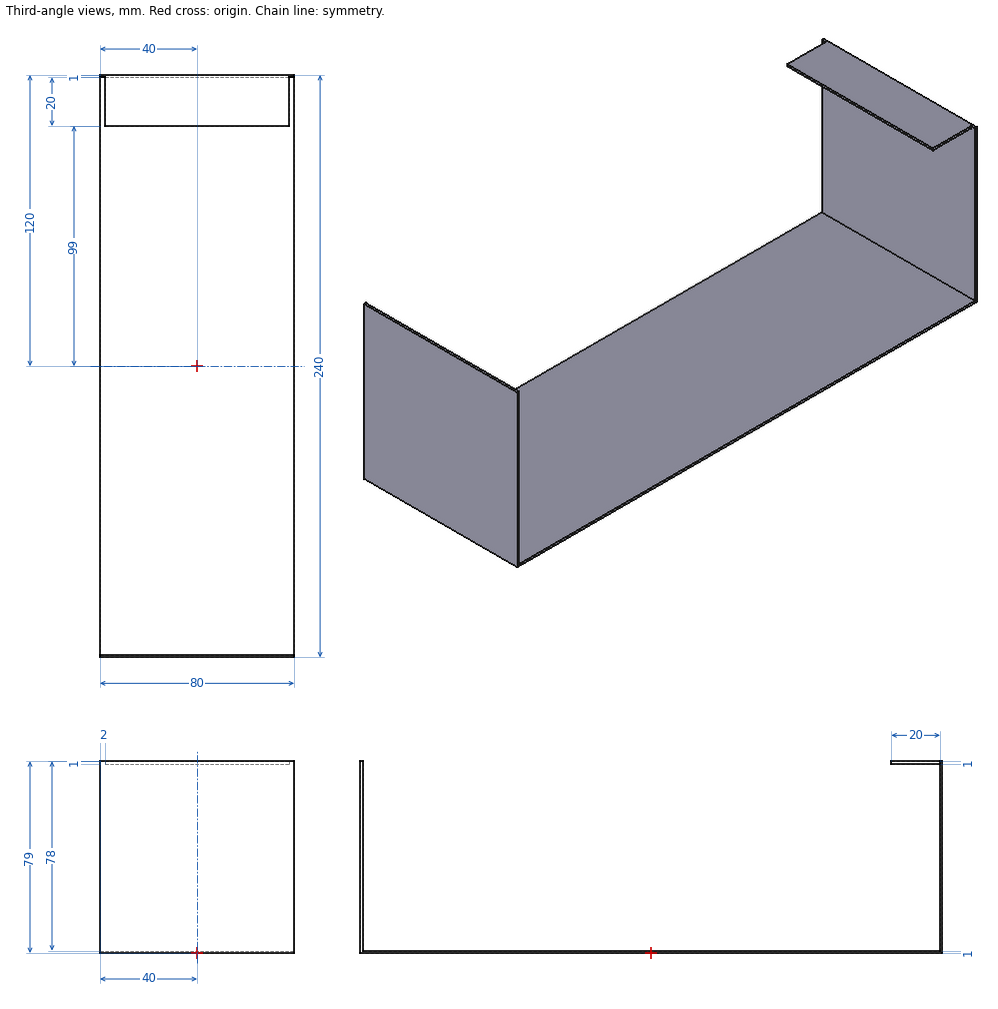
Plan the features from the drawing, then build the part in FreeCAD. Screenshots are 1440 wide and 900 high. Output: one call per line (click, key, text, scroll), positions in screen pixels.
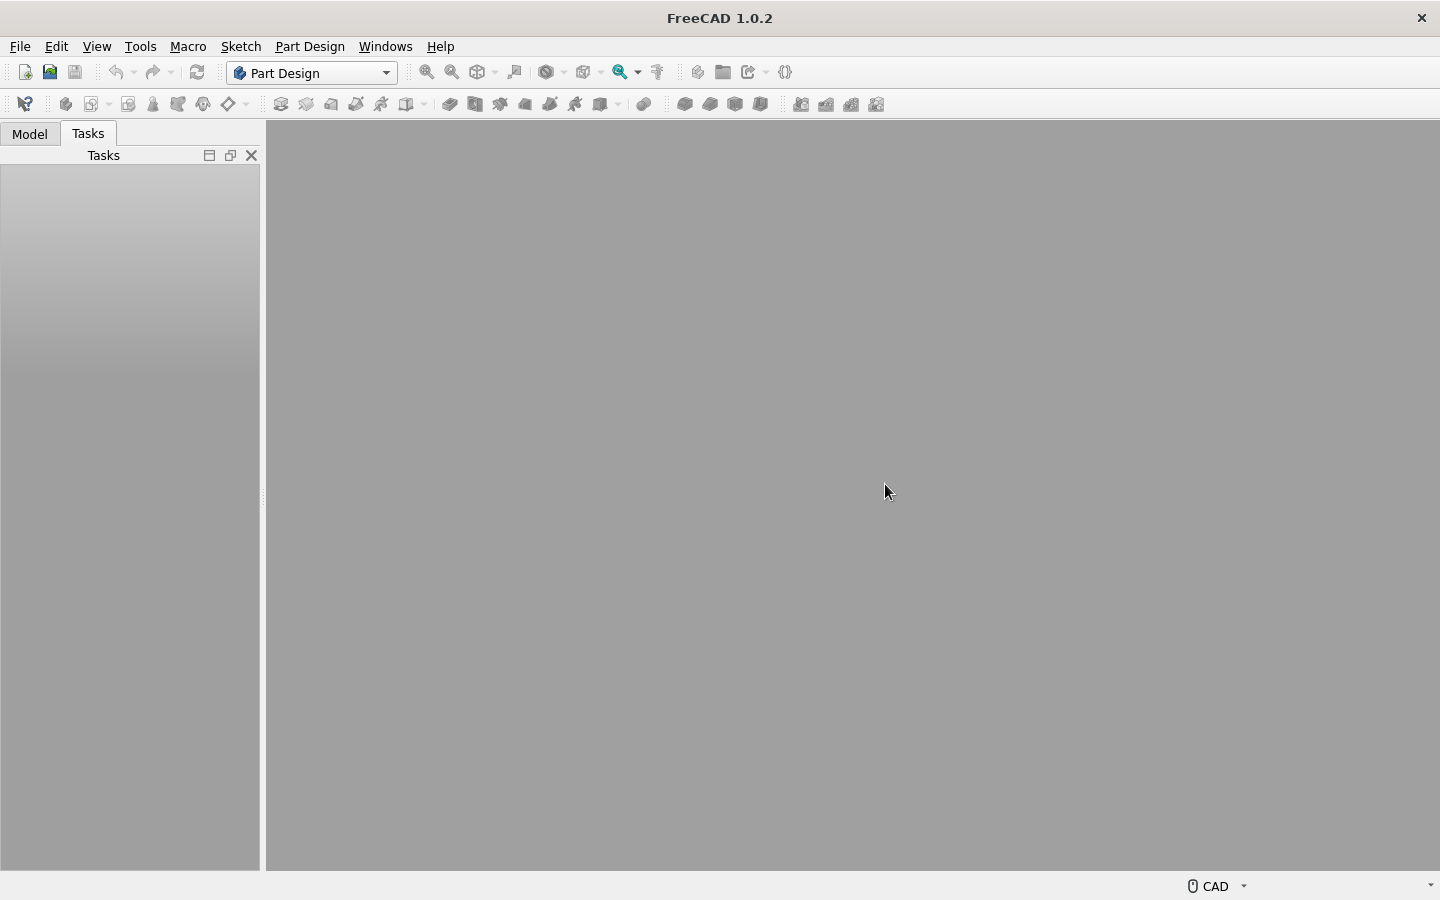
key(ctrl+n)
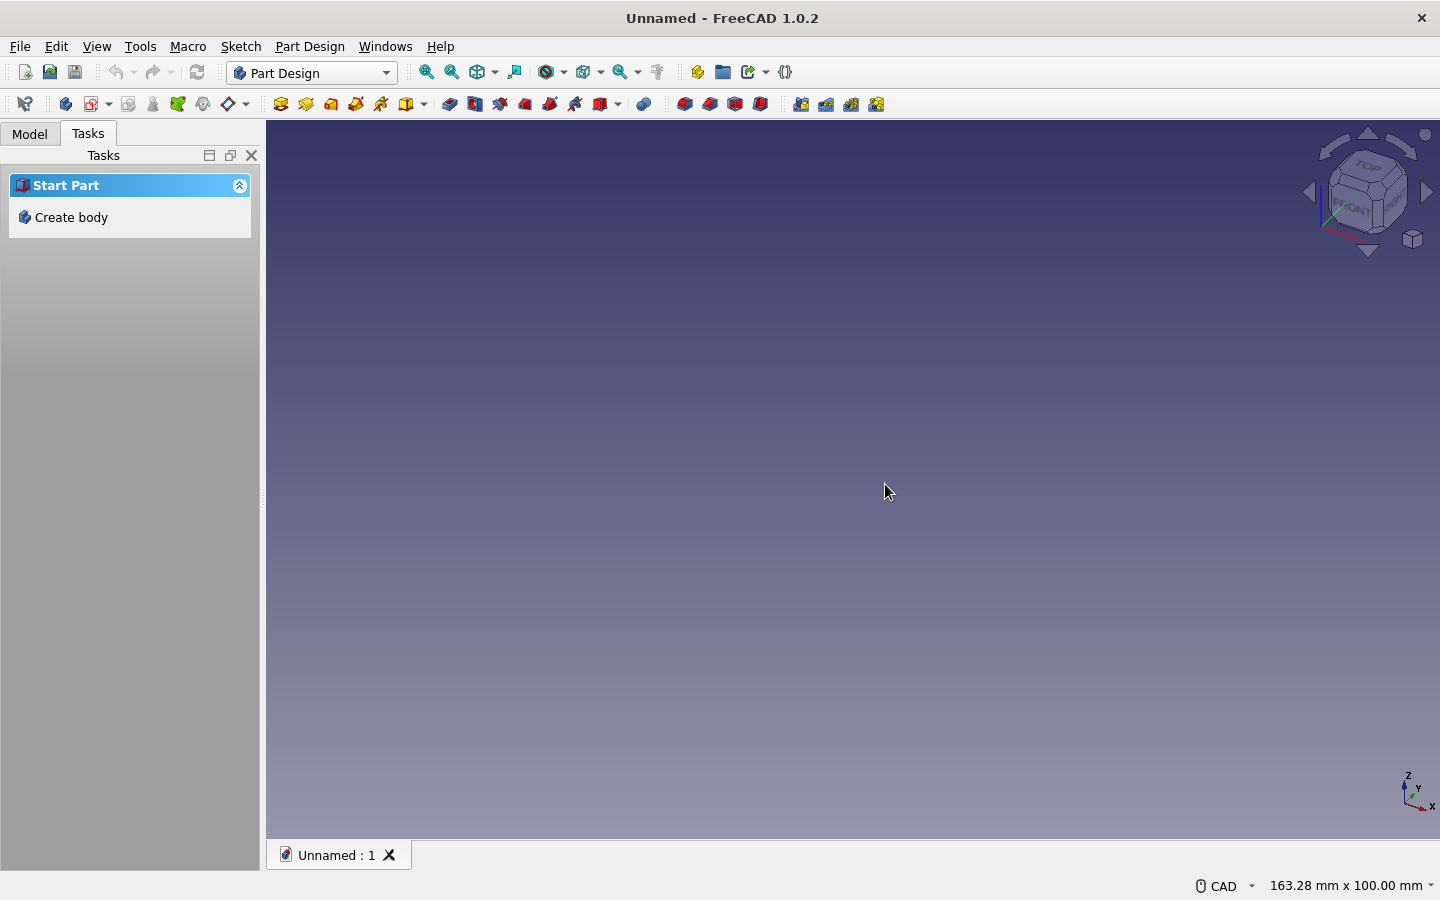
click(90, 104)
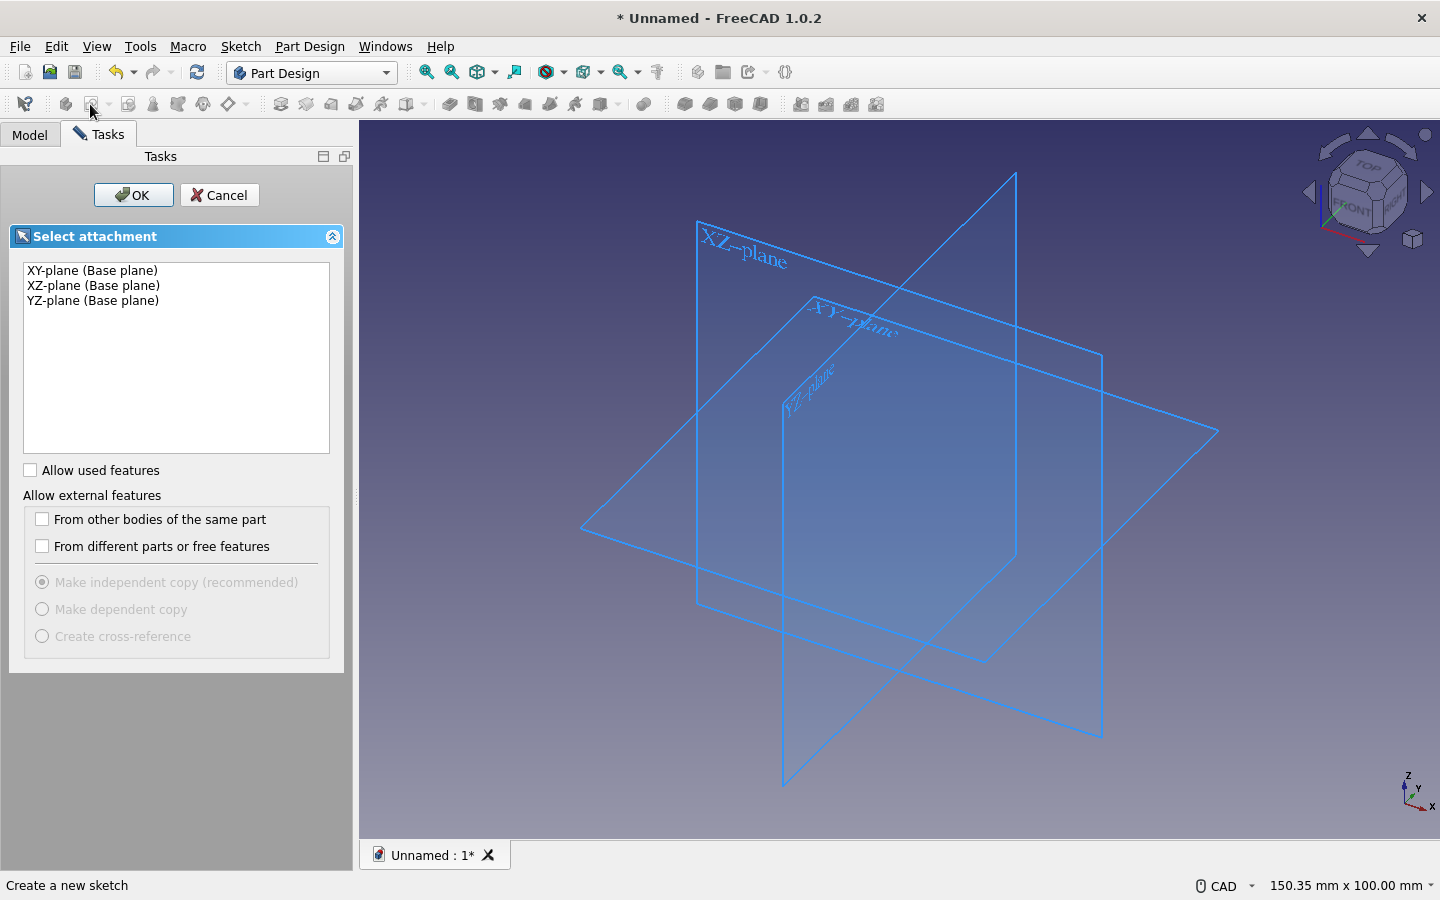
click(84, 270)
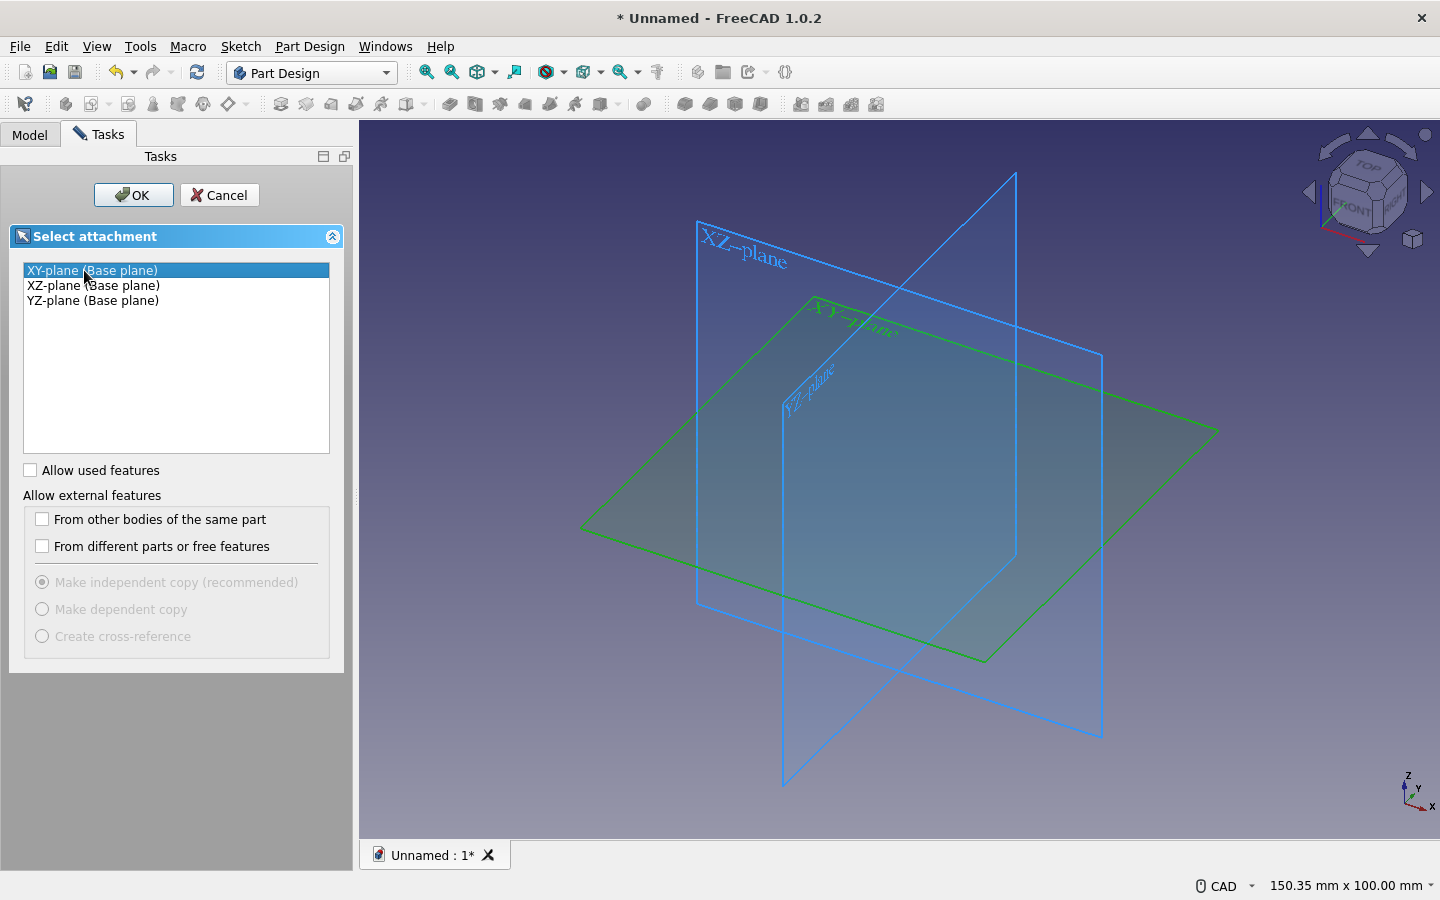
click(134, 195)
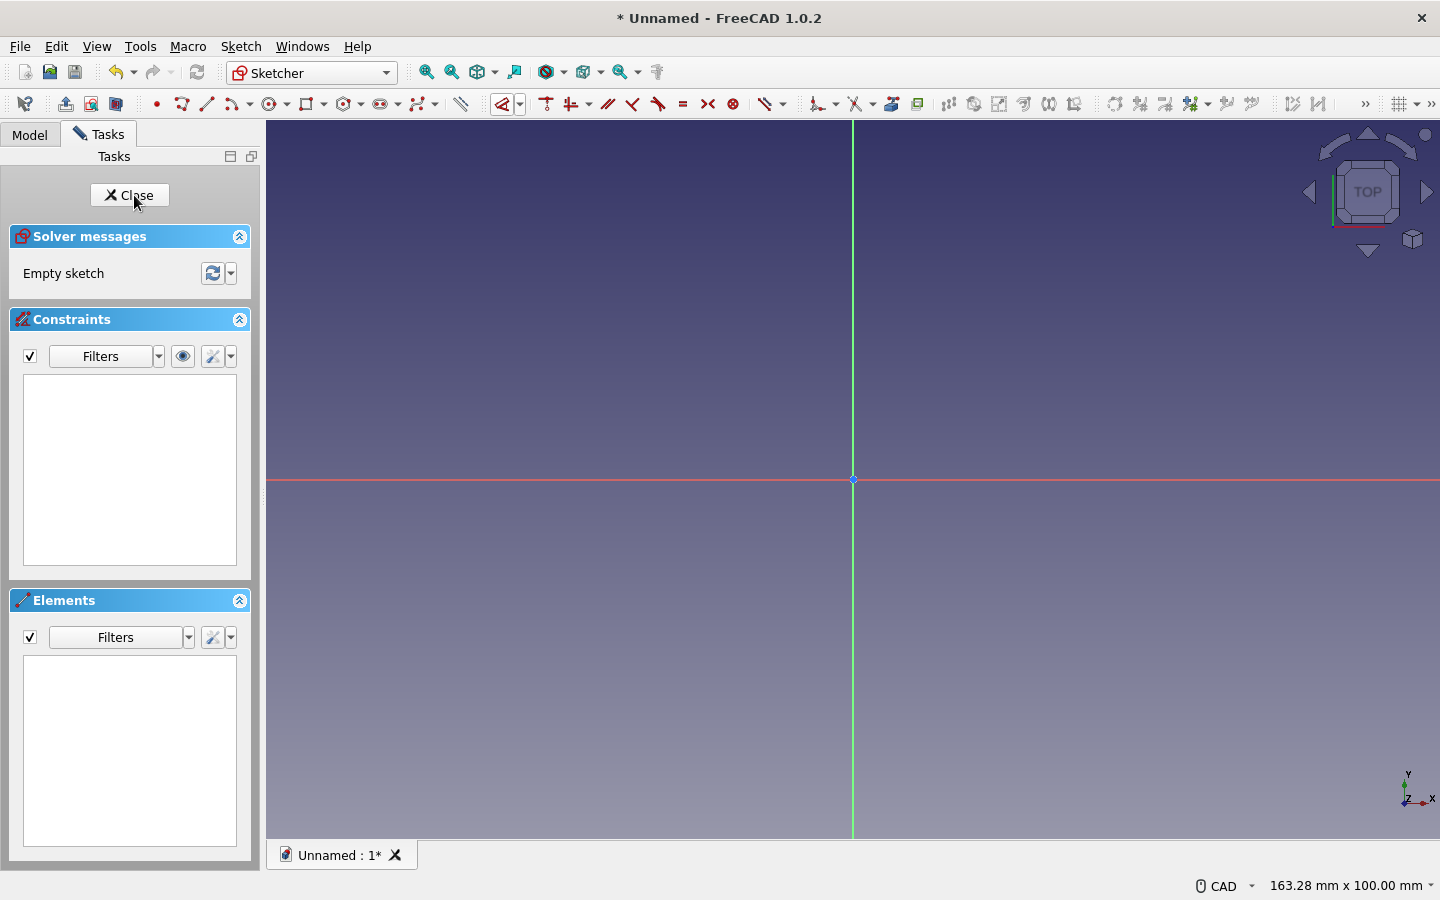
scroll(762, 480, down, 7)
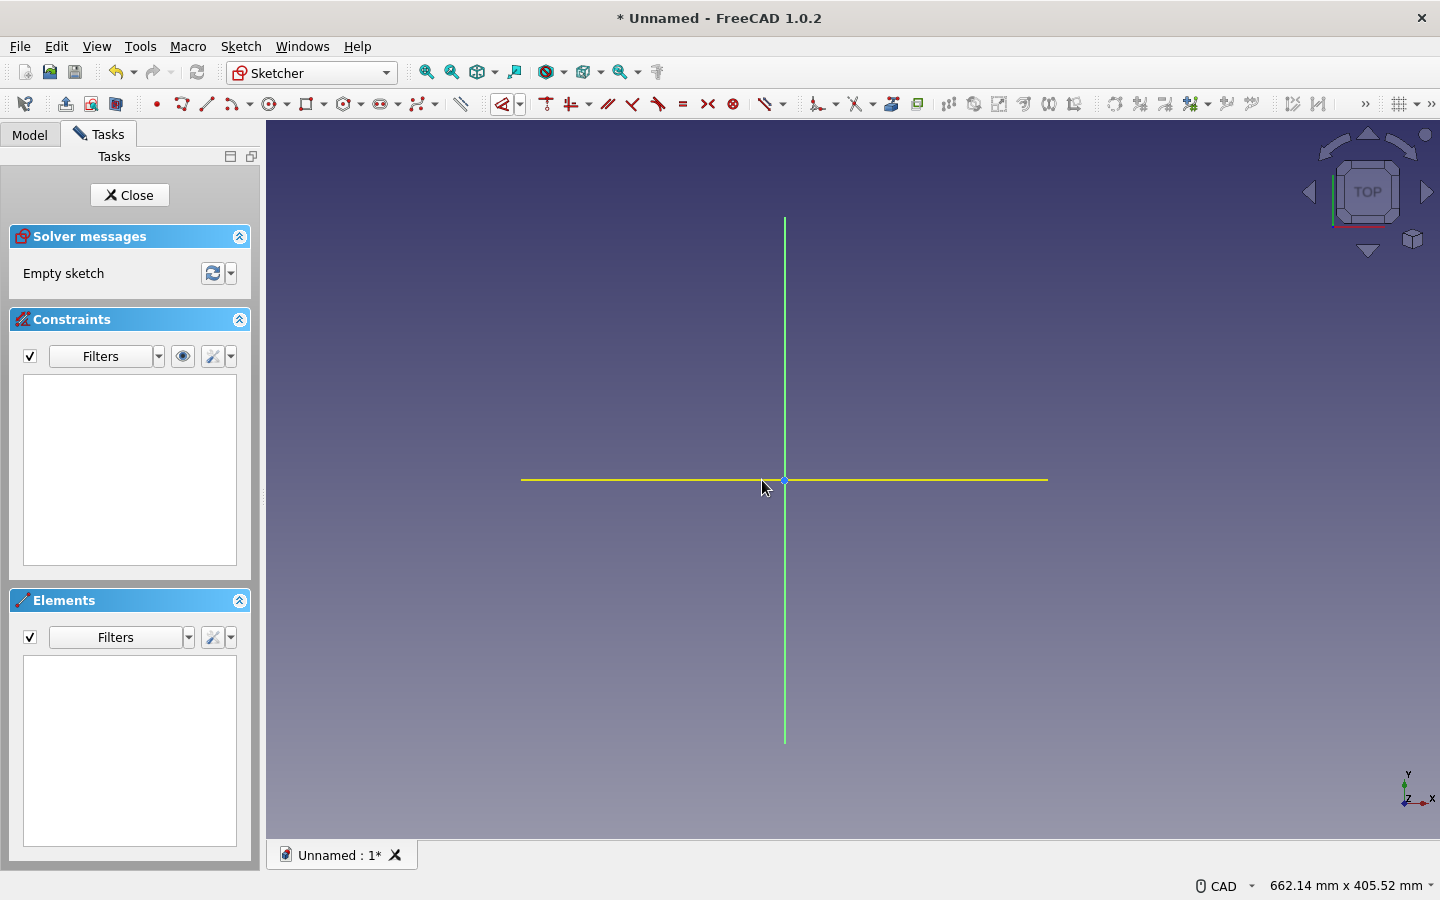
click(324, 104)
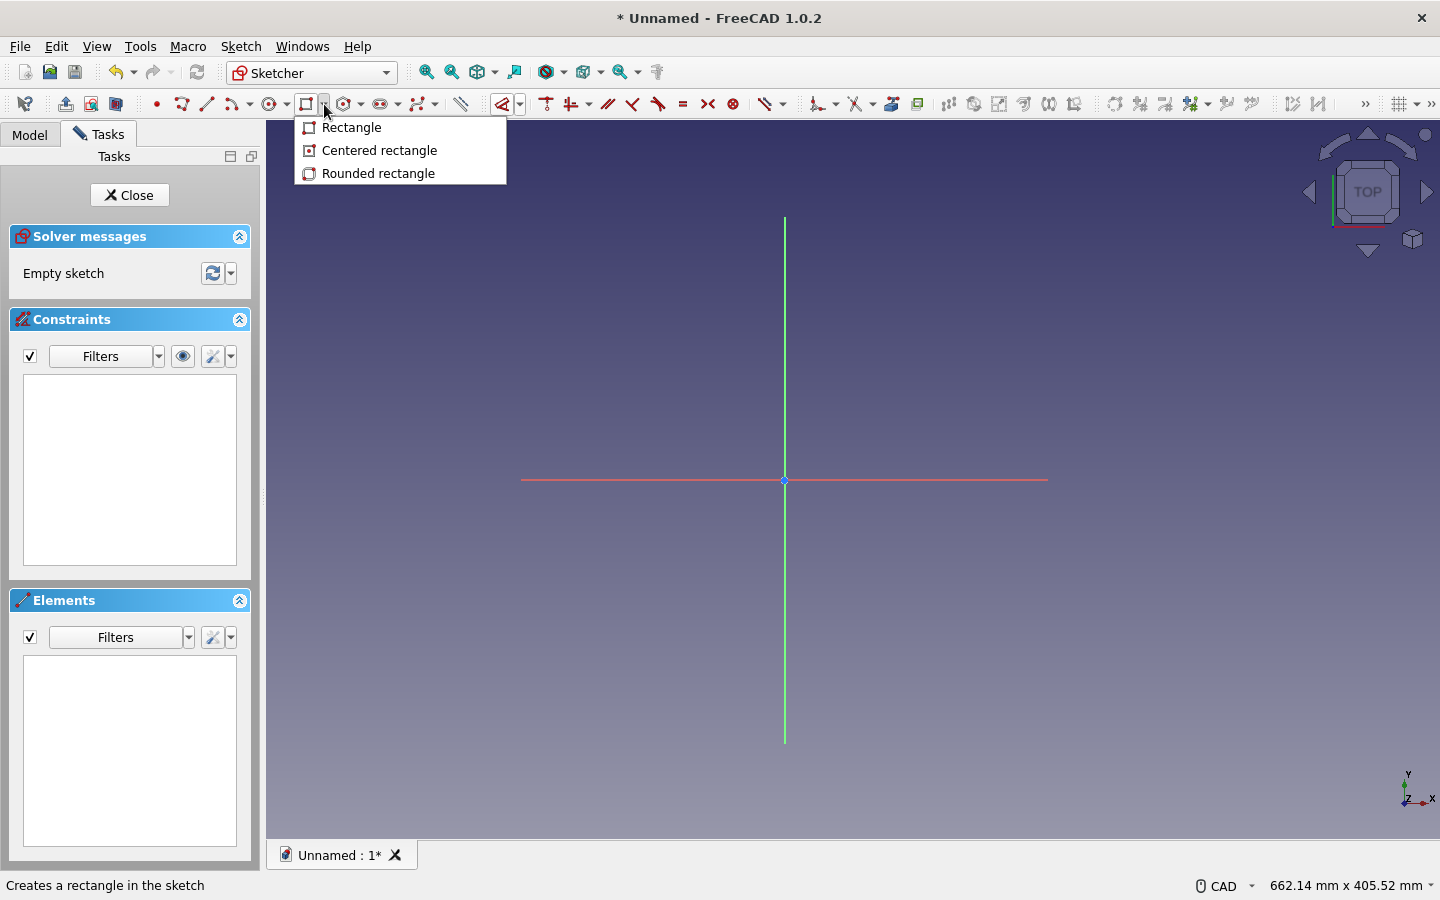
click(400, 150)